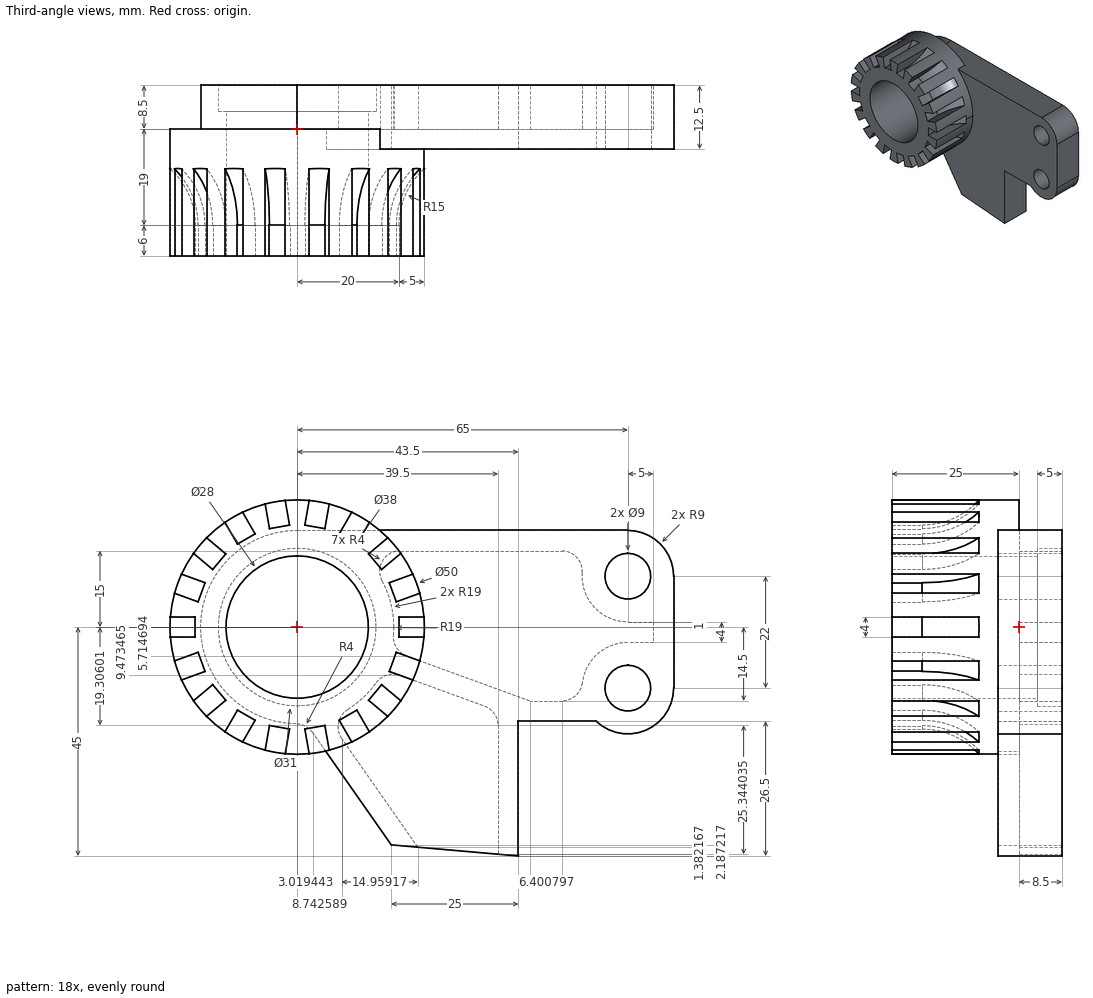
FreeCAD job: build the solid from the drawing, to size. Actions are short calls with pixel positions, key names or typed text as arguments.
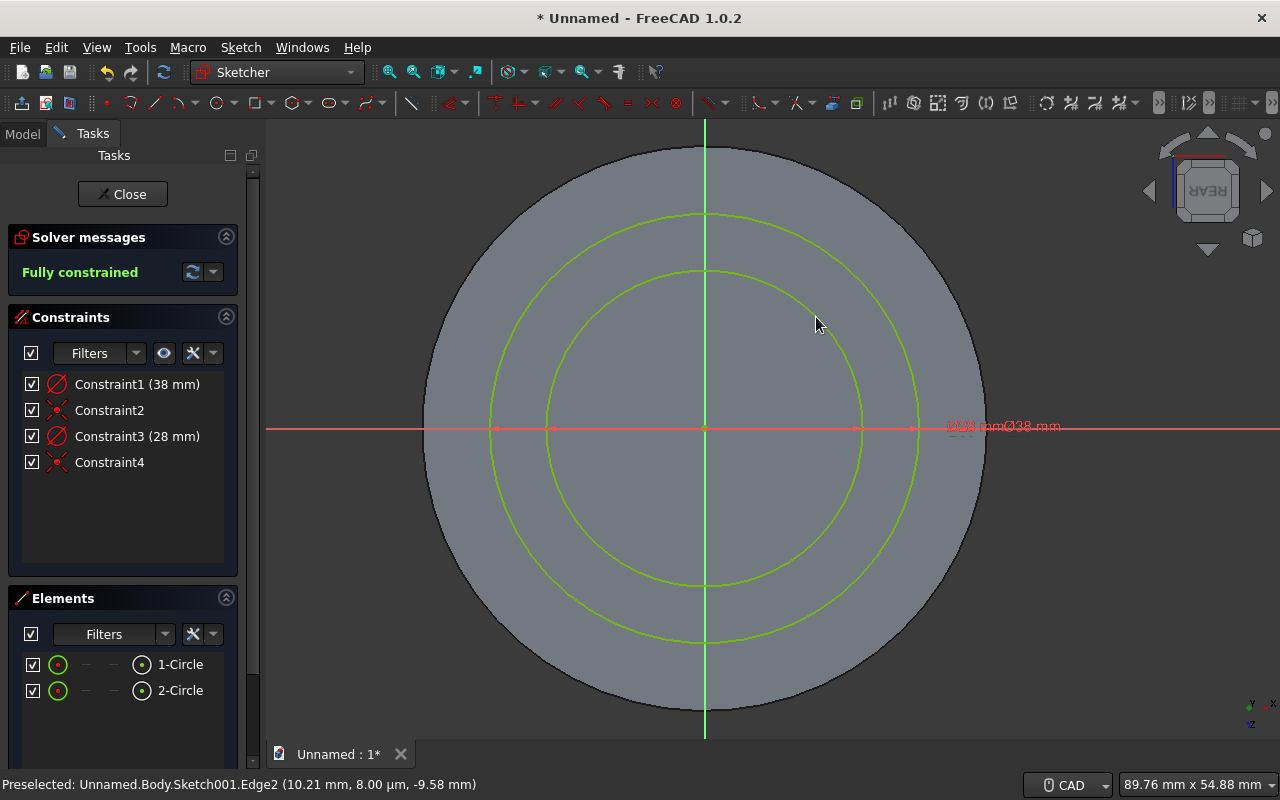
click(123, 194)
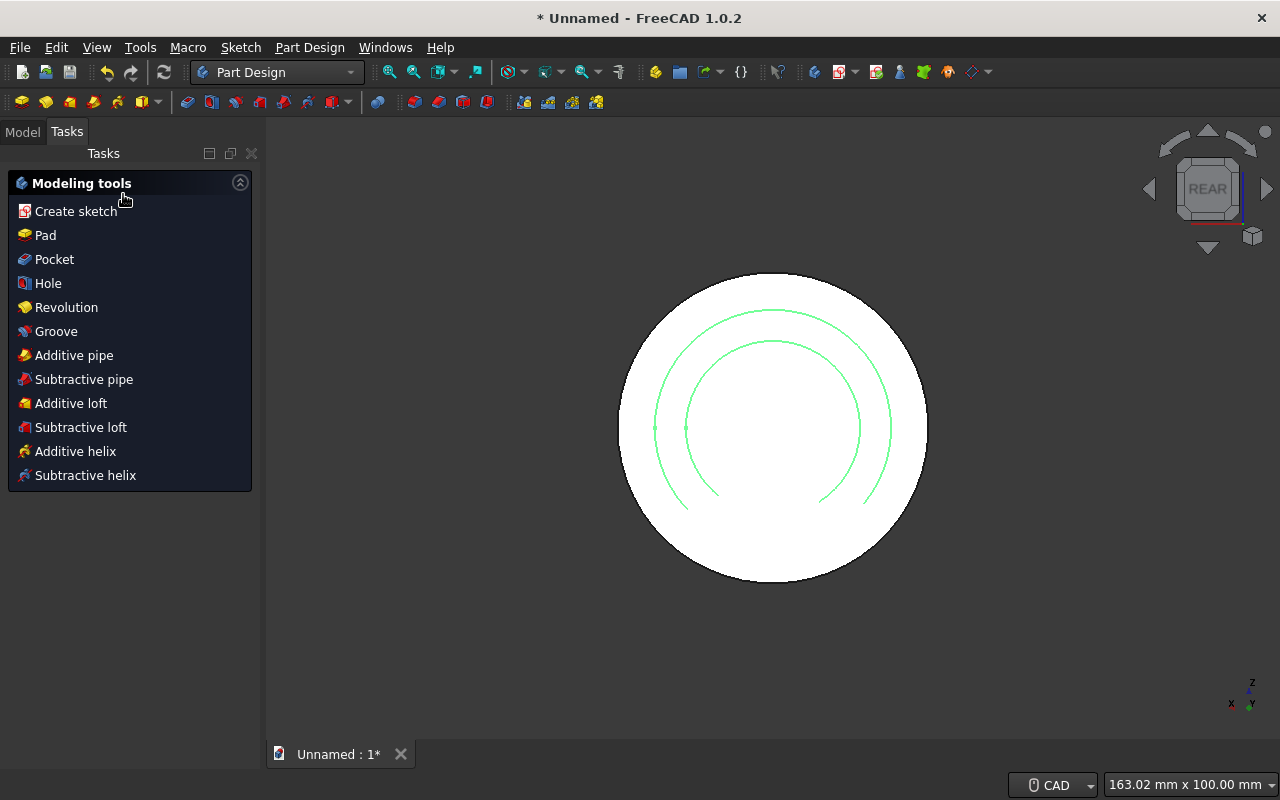
click(22, 102)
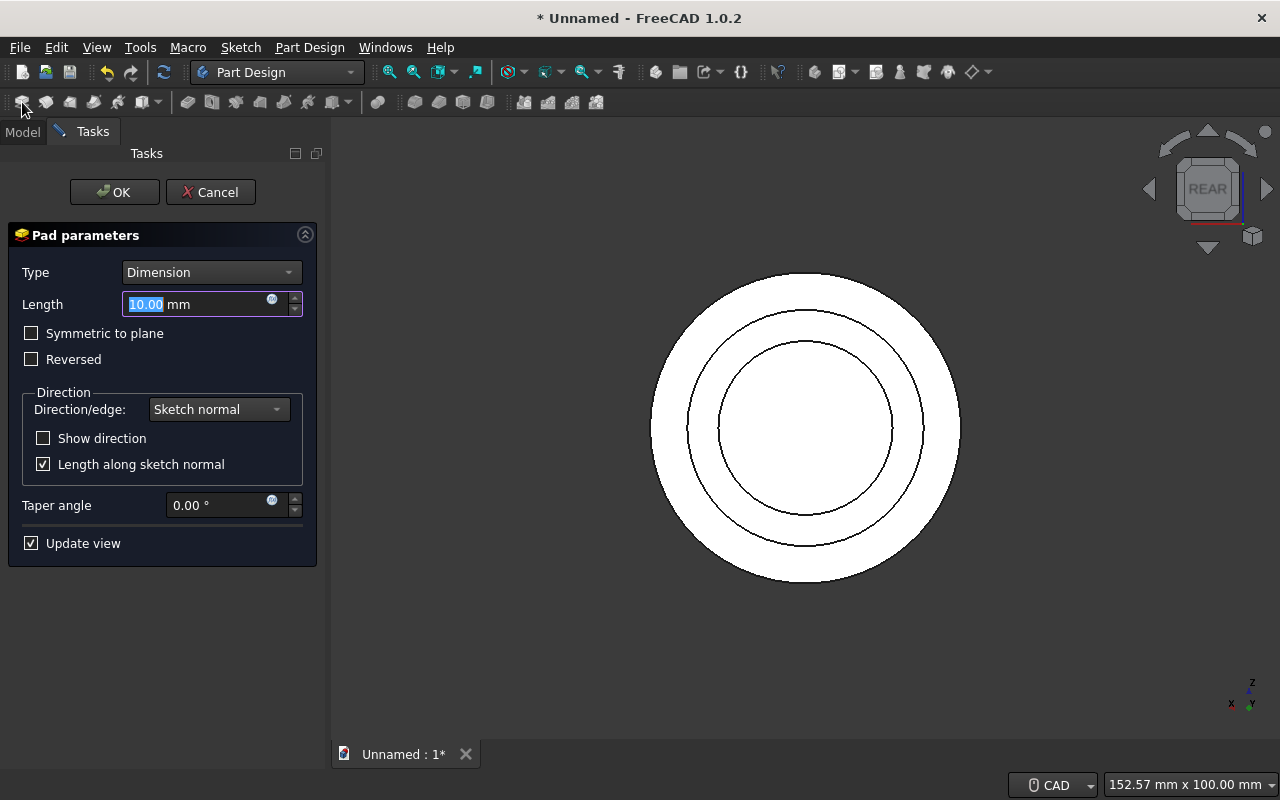
text(8.5)
key(Tab)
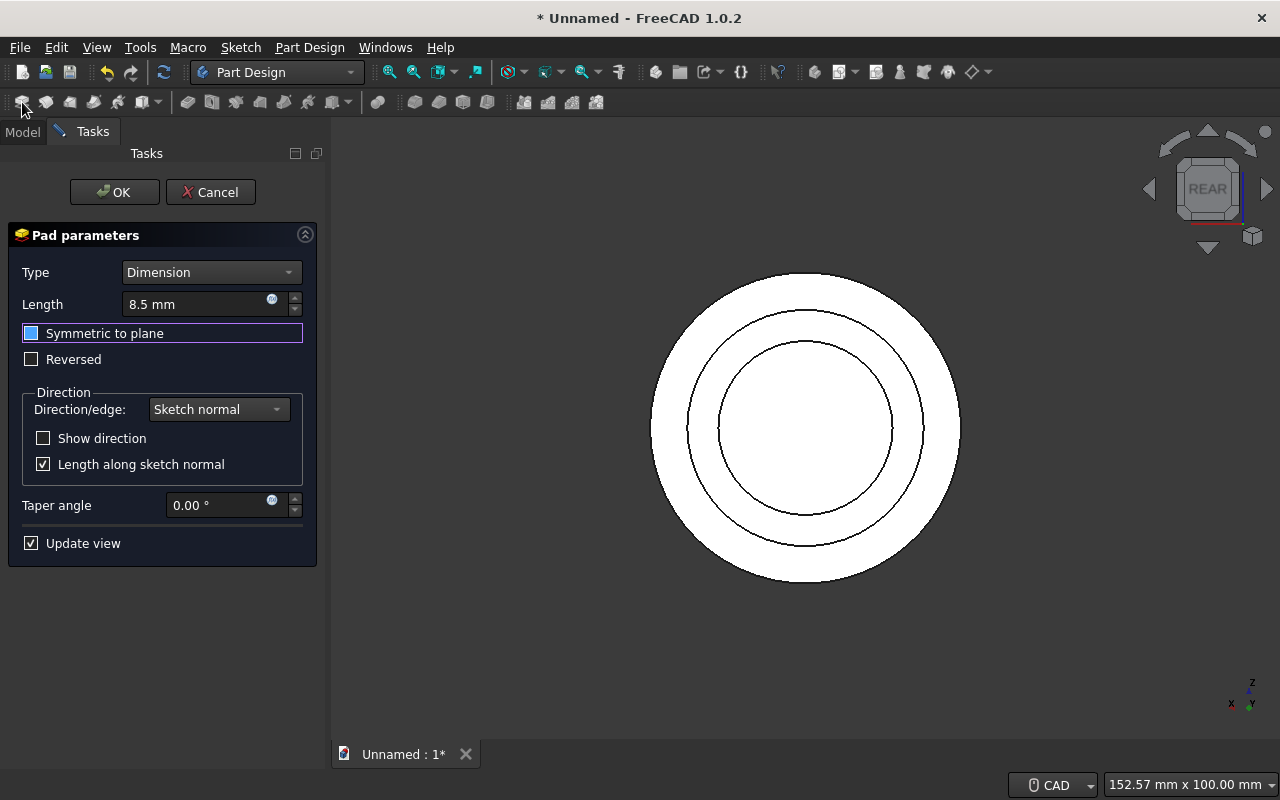
click(115, 192)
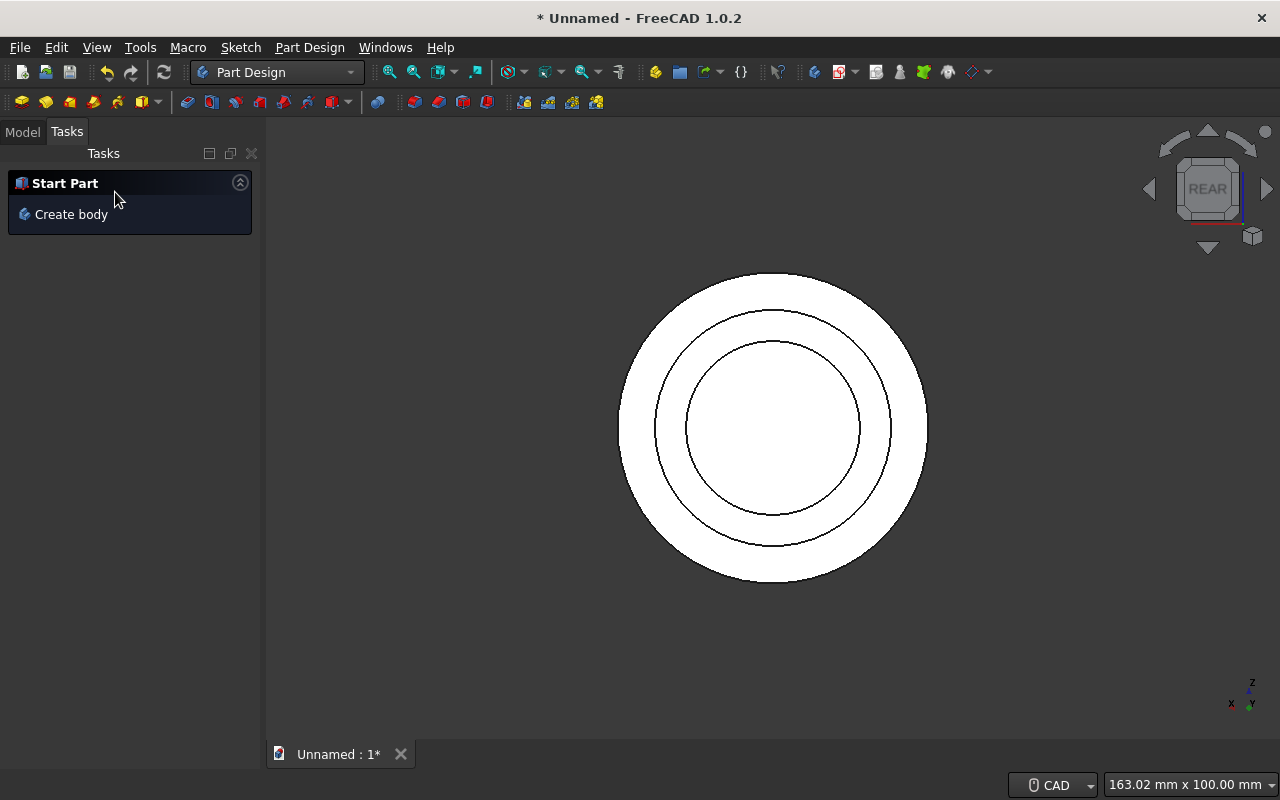
click(640, 427)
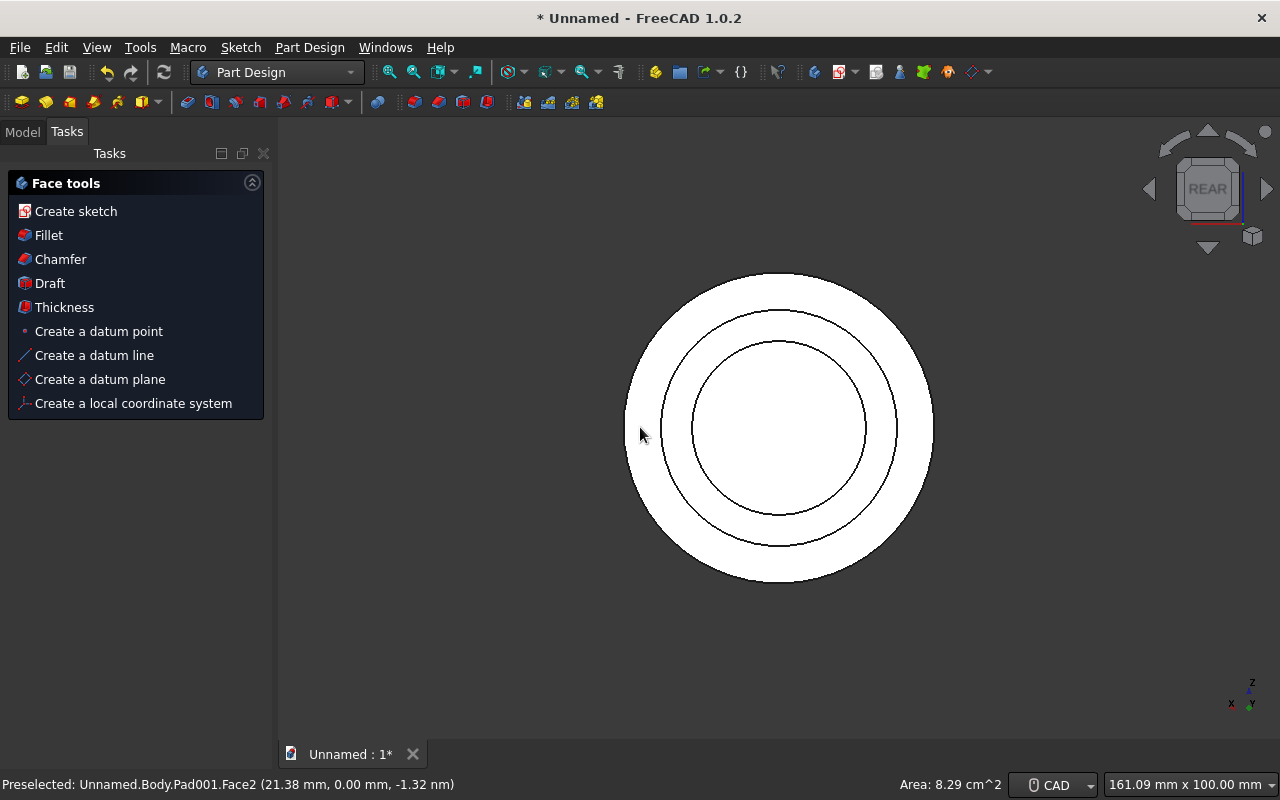
click(840, 72)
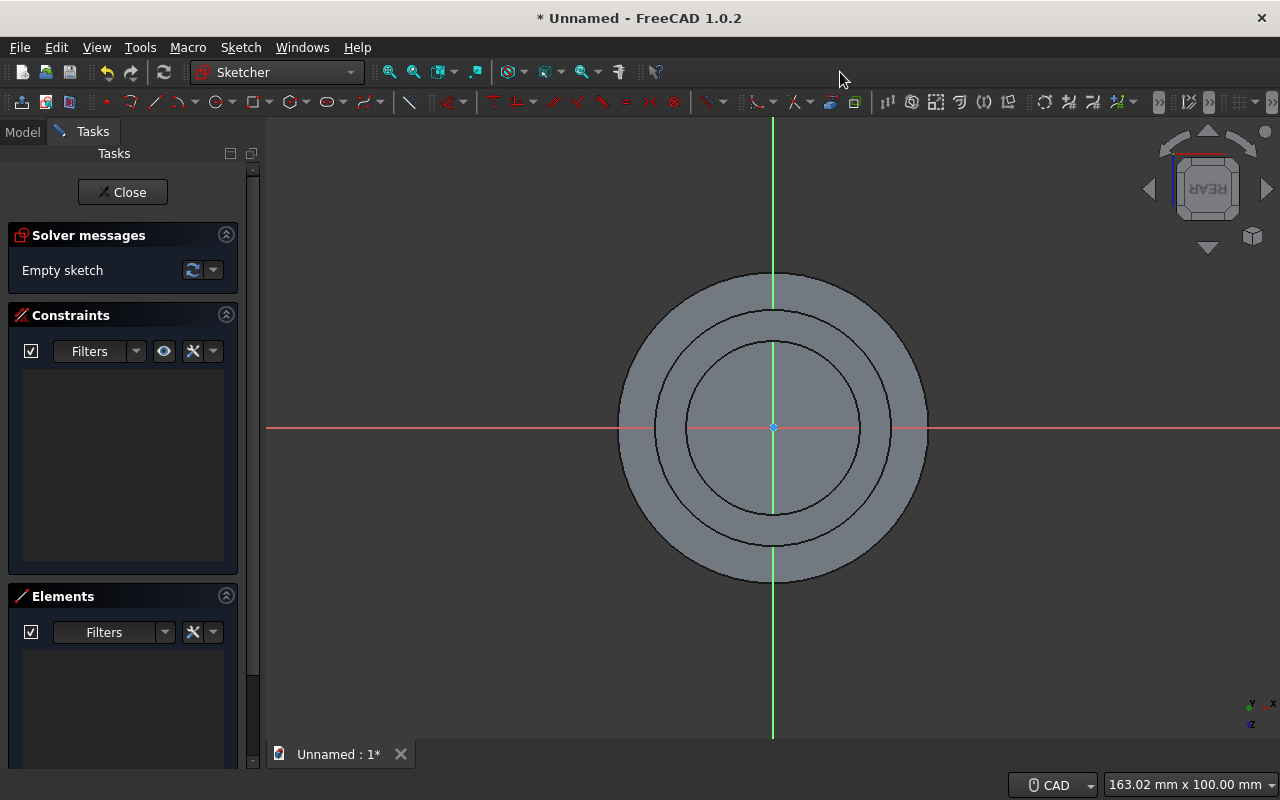
scroll(829, 428, up, 4)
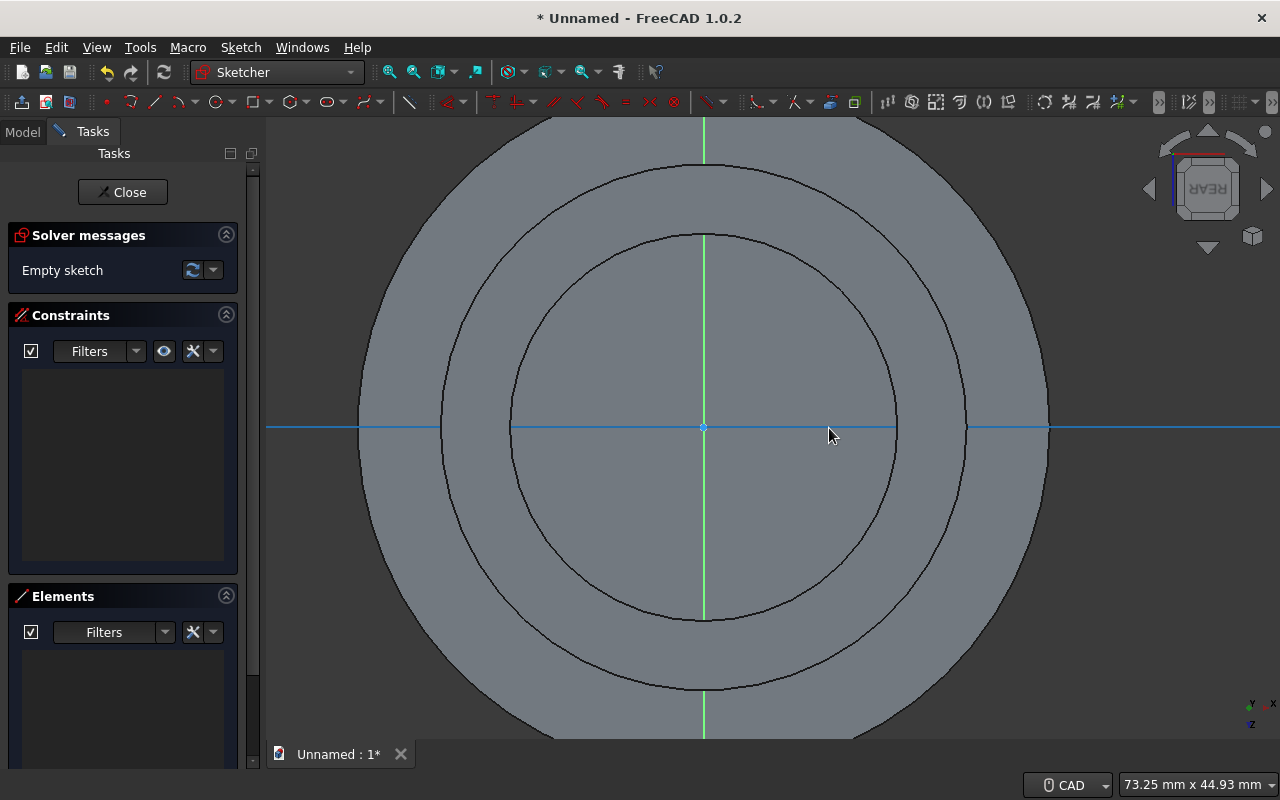
click(216, 102)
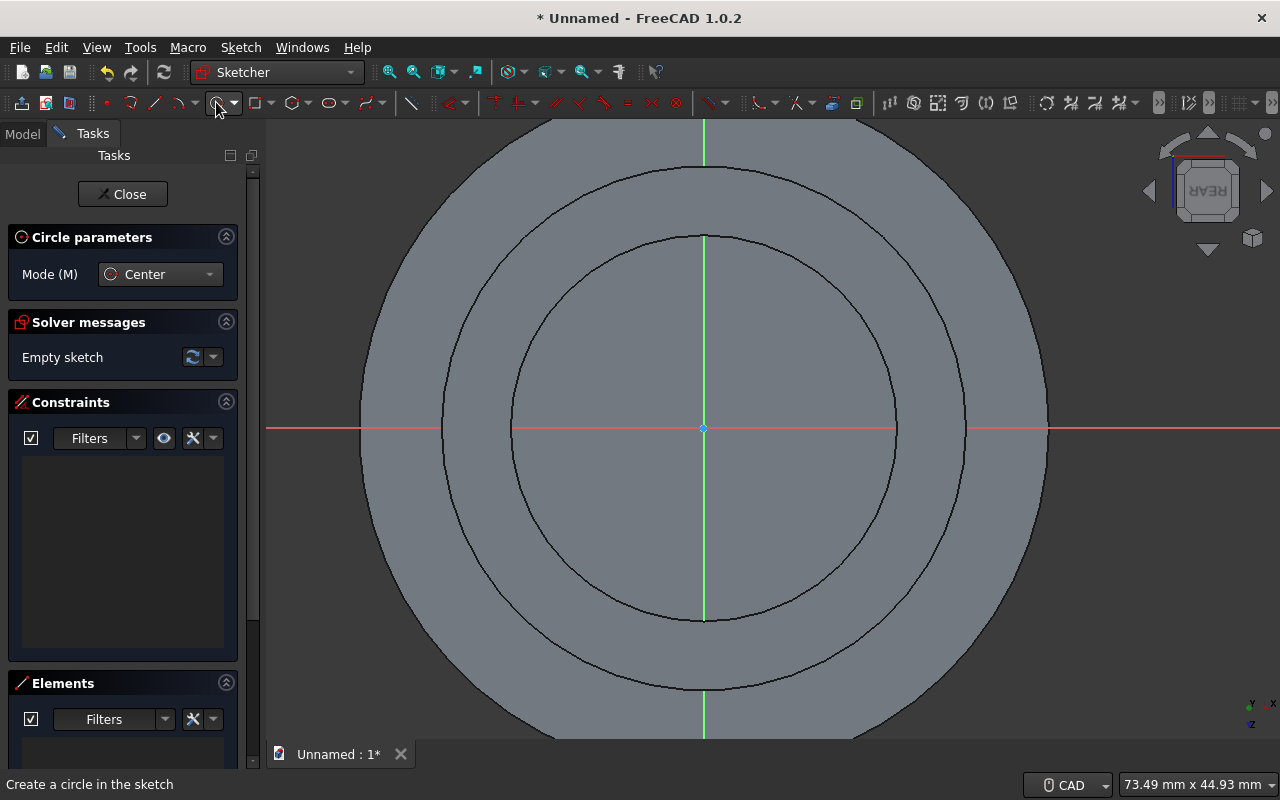
click(704, 428)
move(841, 292)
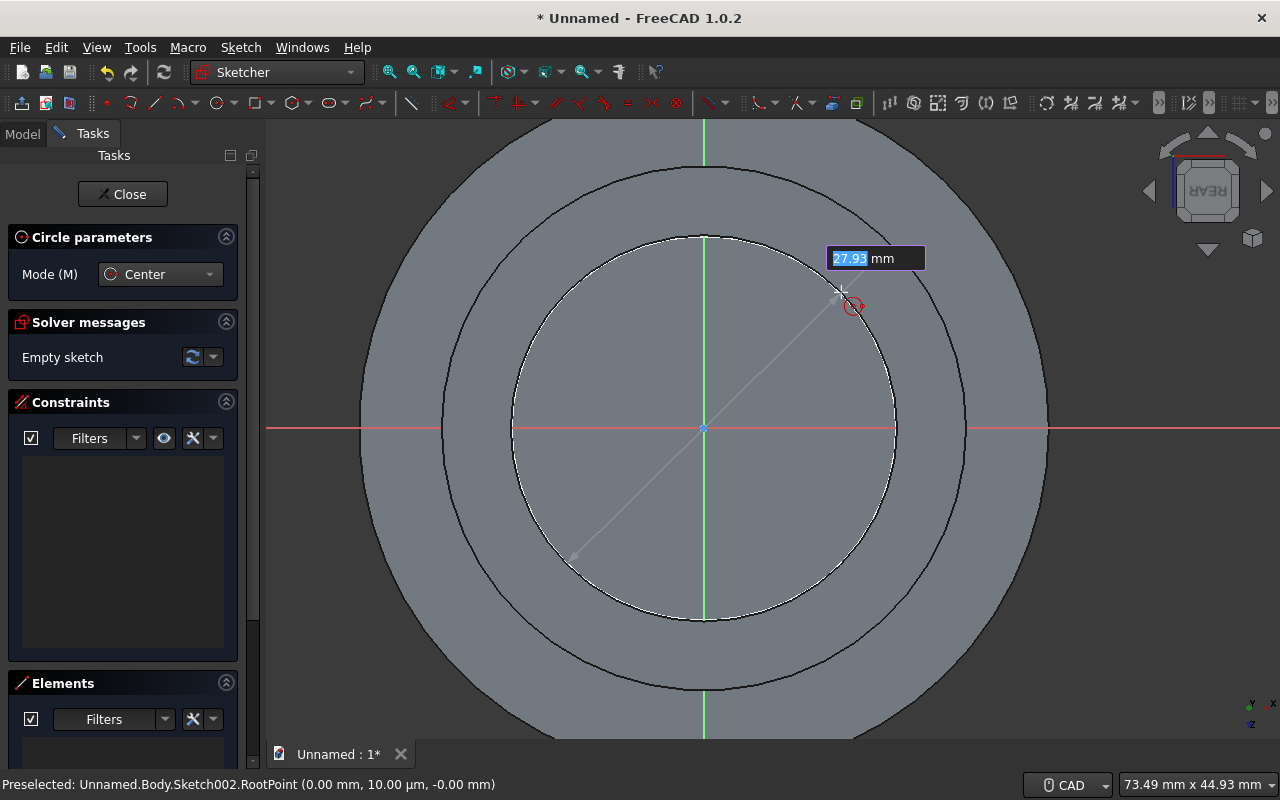
text(28)
key(Return)
key(Escape)